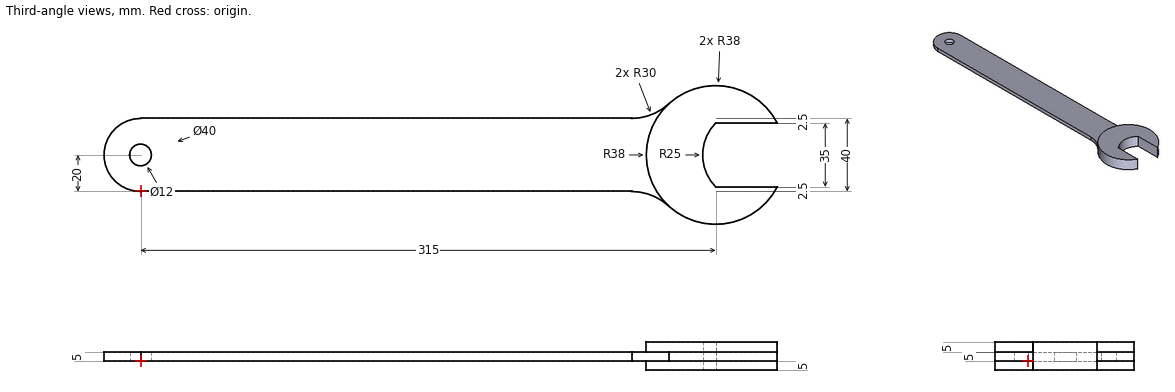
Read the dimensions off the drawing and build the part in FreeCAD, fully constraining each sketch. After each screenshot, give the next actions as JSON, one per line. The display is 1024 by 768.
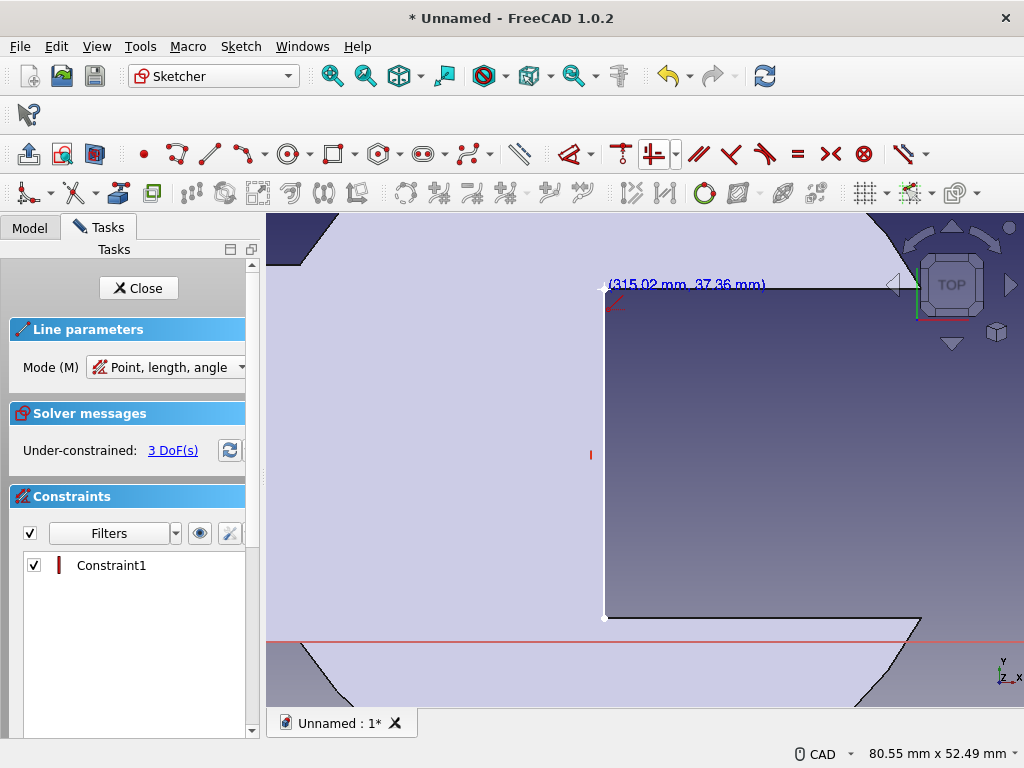
{"action": "left_click", "coordinate": [242, 154]}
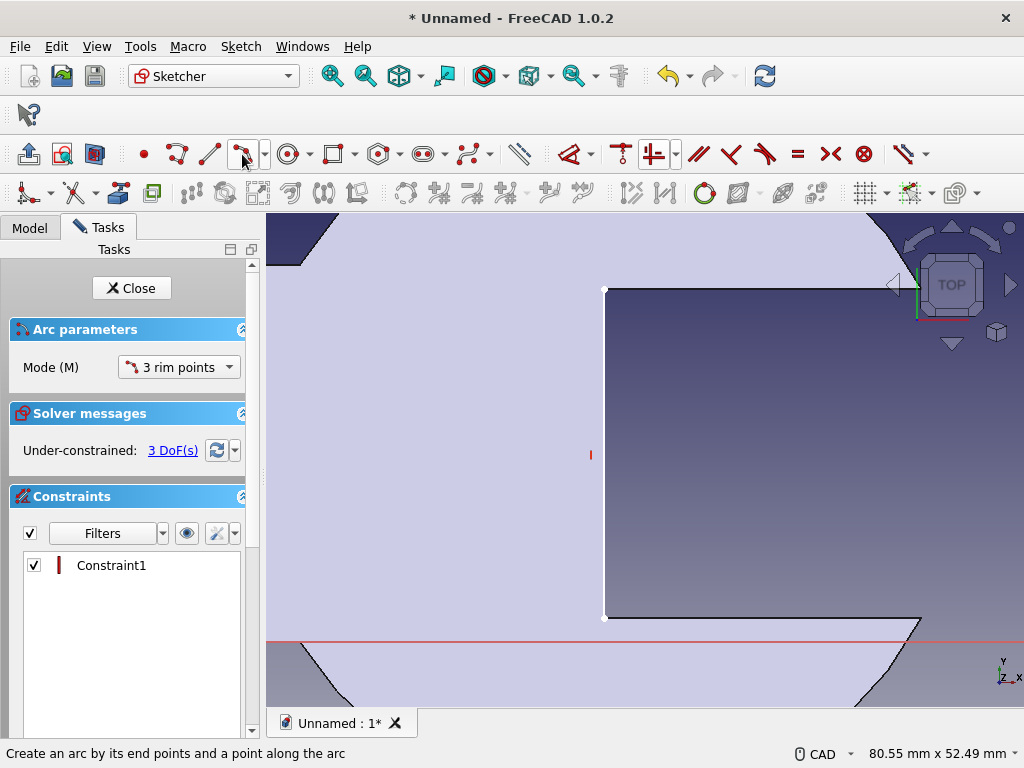
{"action": "left_click", "coordinate": [604, 290]}
{"action": "left_click", "coordinate": [604, 619]}
{"action": "left_click", "coordinate": [537, 453]}
{"action": "key", "text": "Escape"}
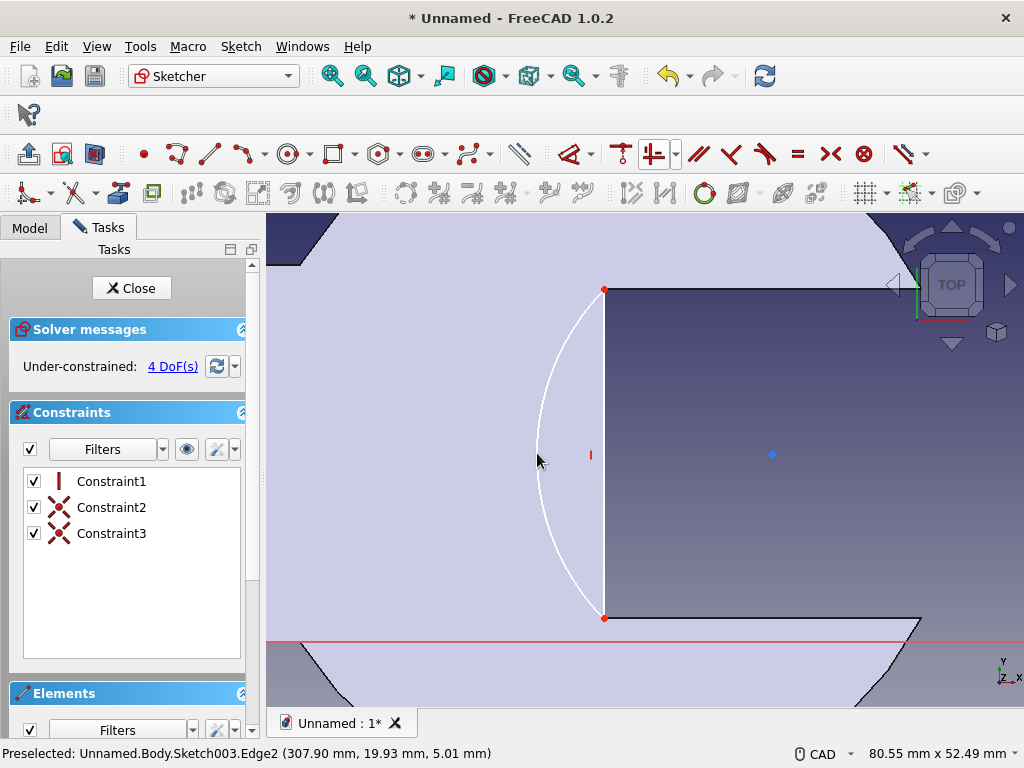
{"action": "left_click", "coordinate": [568, 154]}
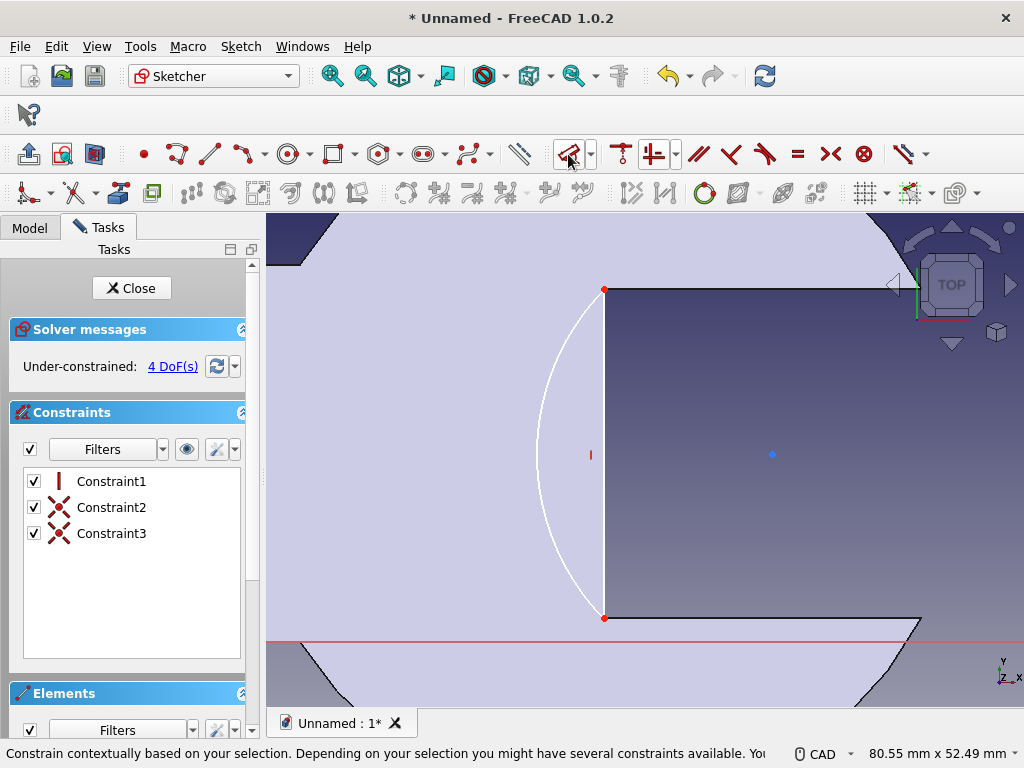
{"action": "left_click", "coordinate": [548, 383]}
{"action": "left_click", "coordinate": [518, 373]}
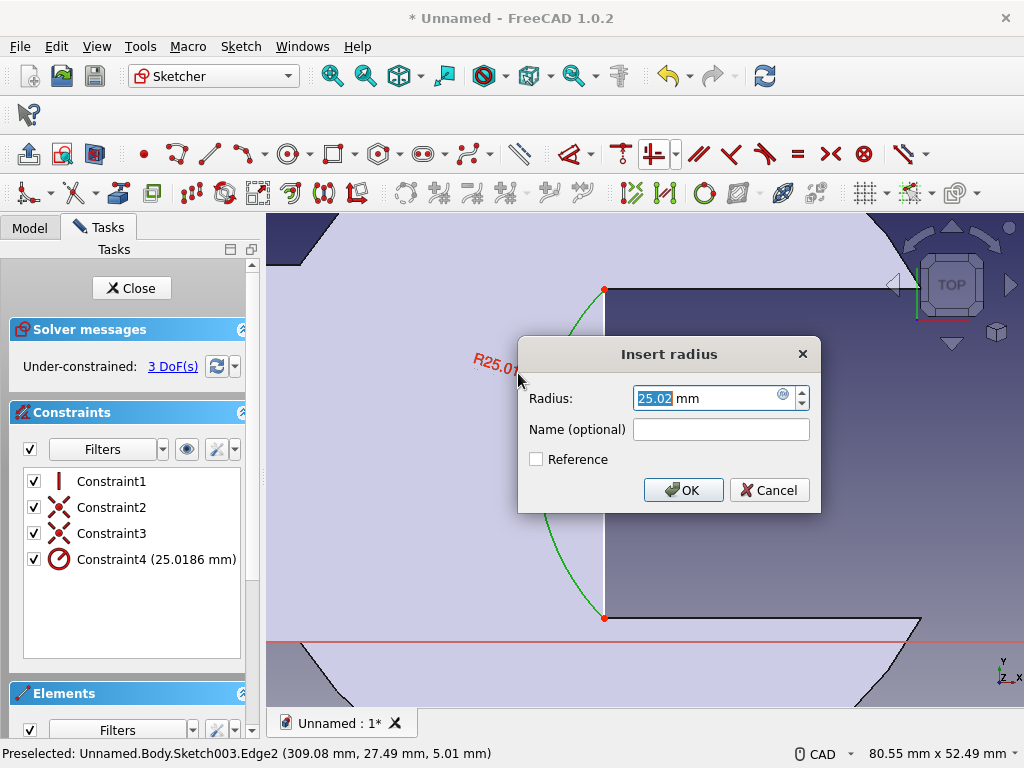
{"action": "type", "text": "25"}
{"action": "key", "text": "Return"}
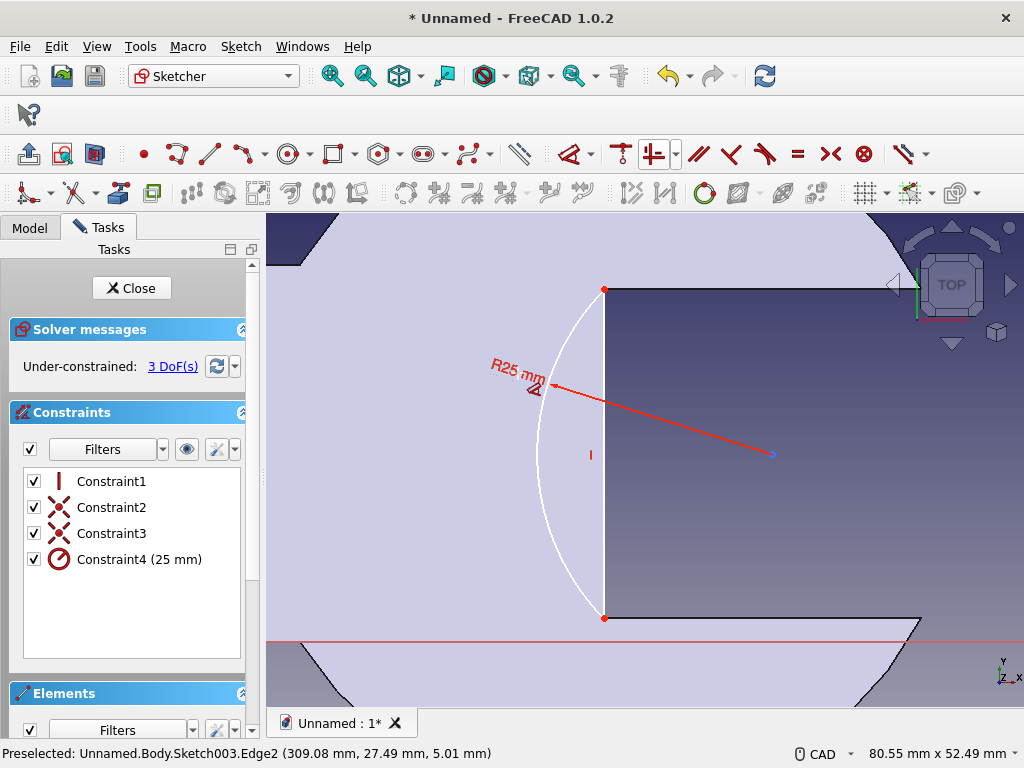
{"action": "left_click", "coordinate": [604, 520]}
{"action": "left_click", "coordinate": [638, 454]}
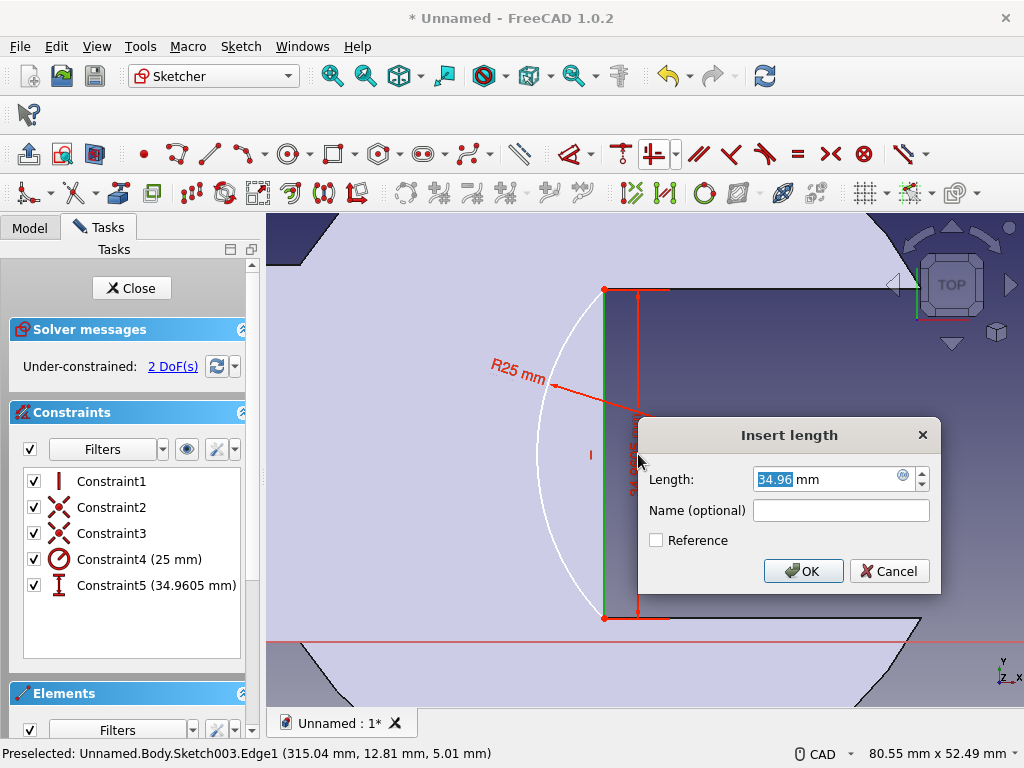
{"action": "type", "text": "35"}
{"action": "key", "text": "Return"}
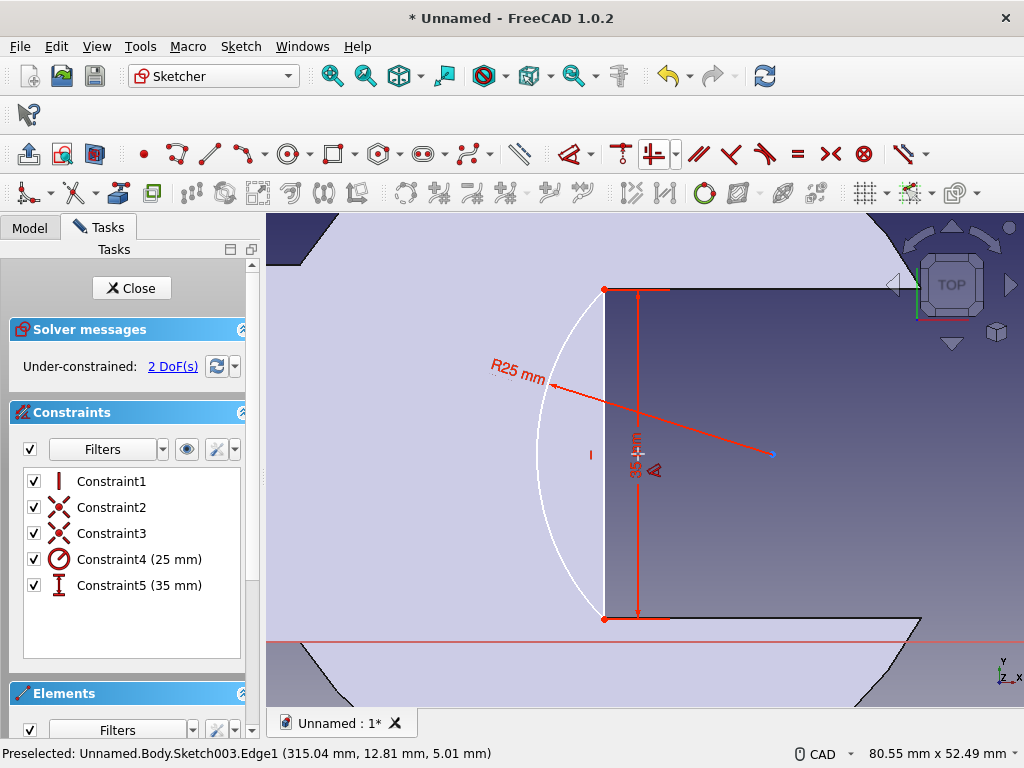
{"action": "left_click", "coordinate": [772, 455]}
{"action": "left_click", "coordinate": [806, 548]}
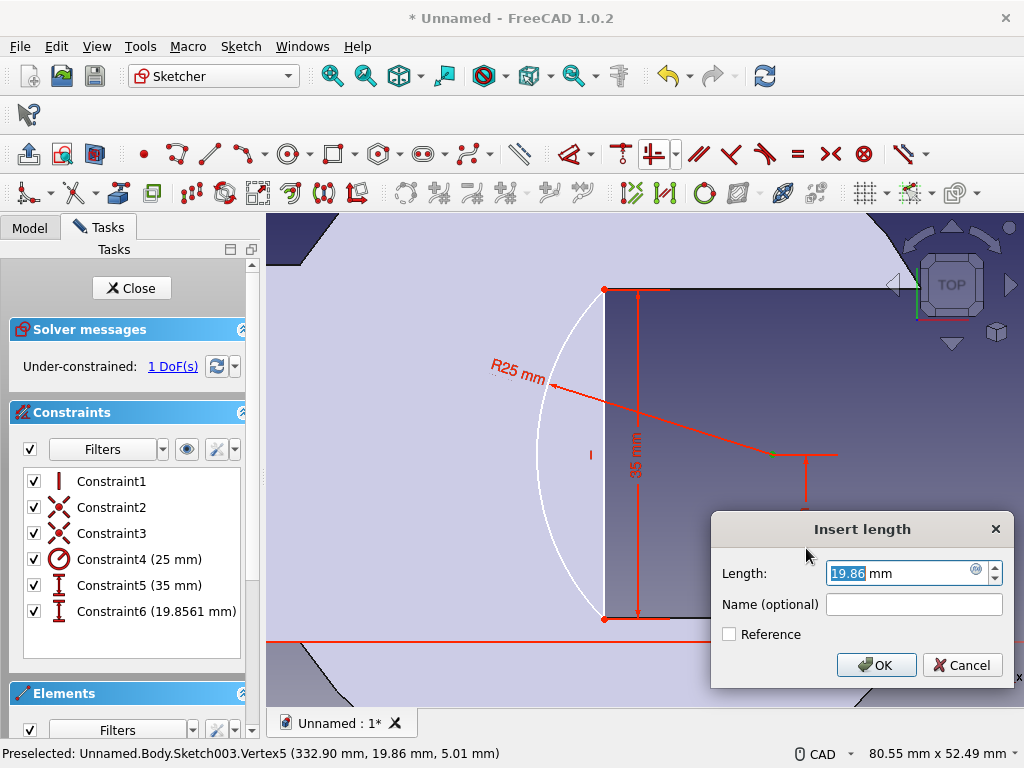
{"action": "type", "text": "20"}
{"action": "key", "text": "Return"}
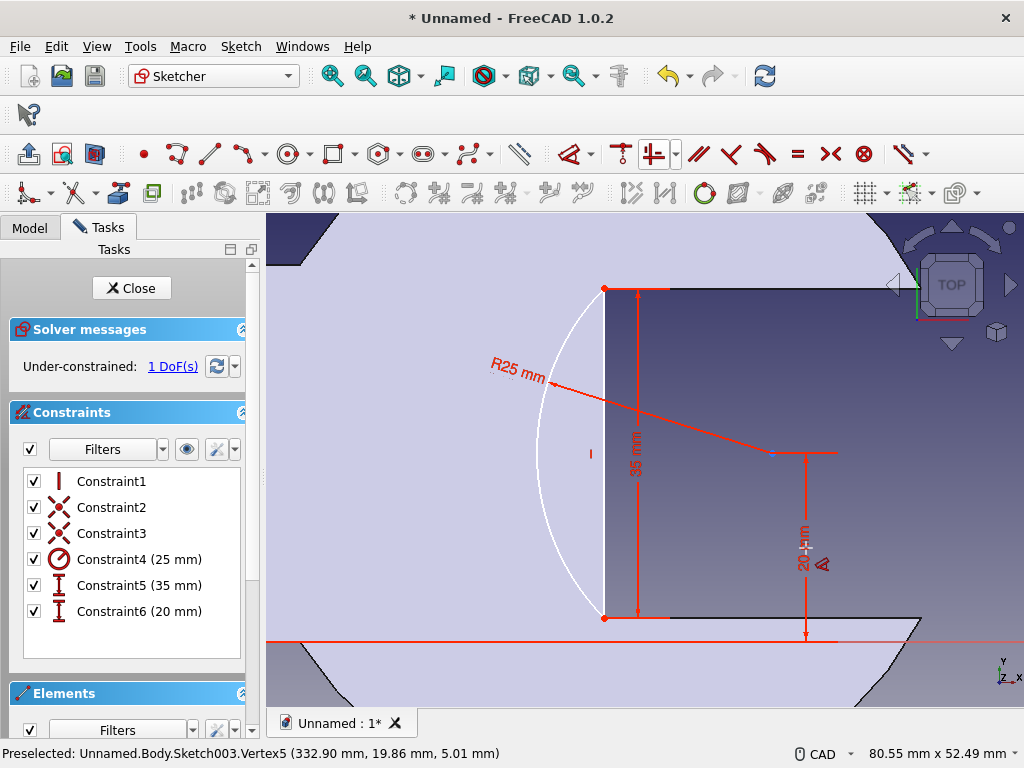
{"action": "left_click", "coordinate": [604, 618]}
{"action": "left_click", "coordinate": [449, 676]}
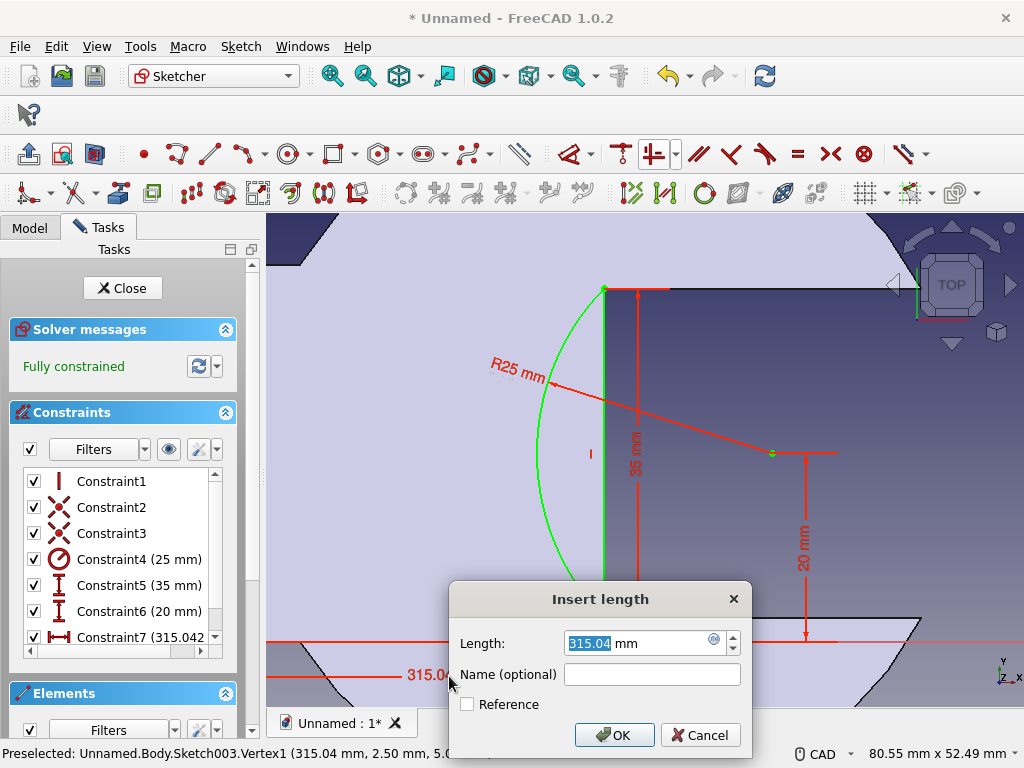
{"action": "type", "text": "315"}
{"action": "key", "text": "Return"}
{"action": "key", "text": "Escape"}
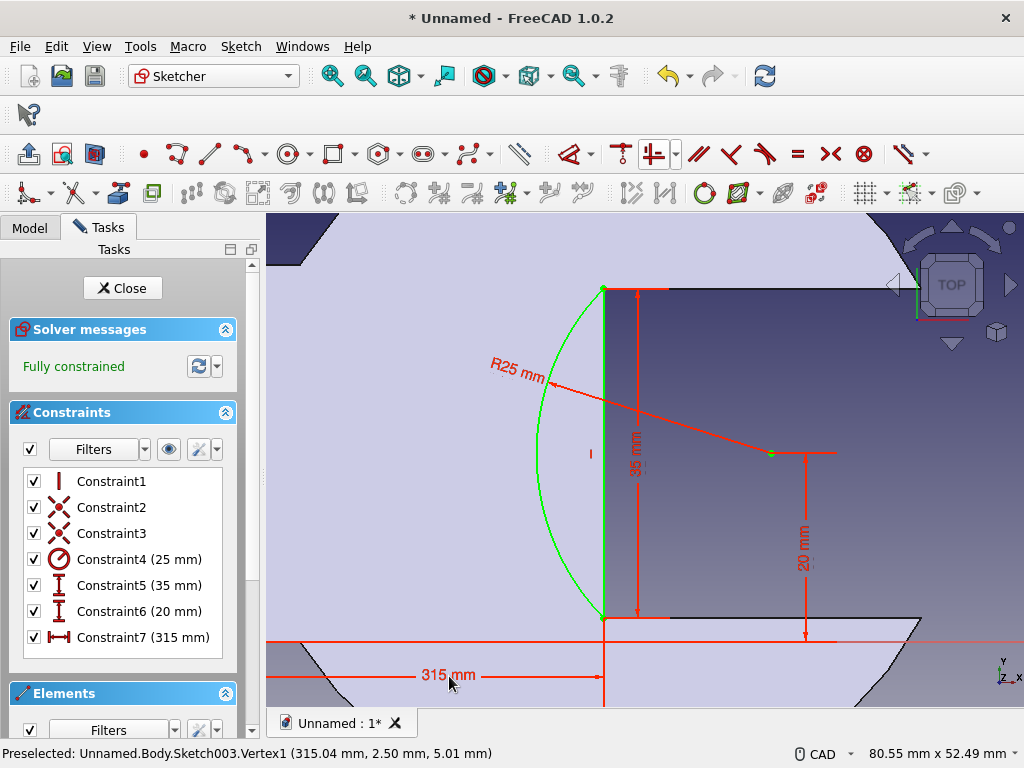
{"action": "left_click", "coordinate": [123, 288]}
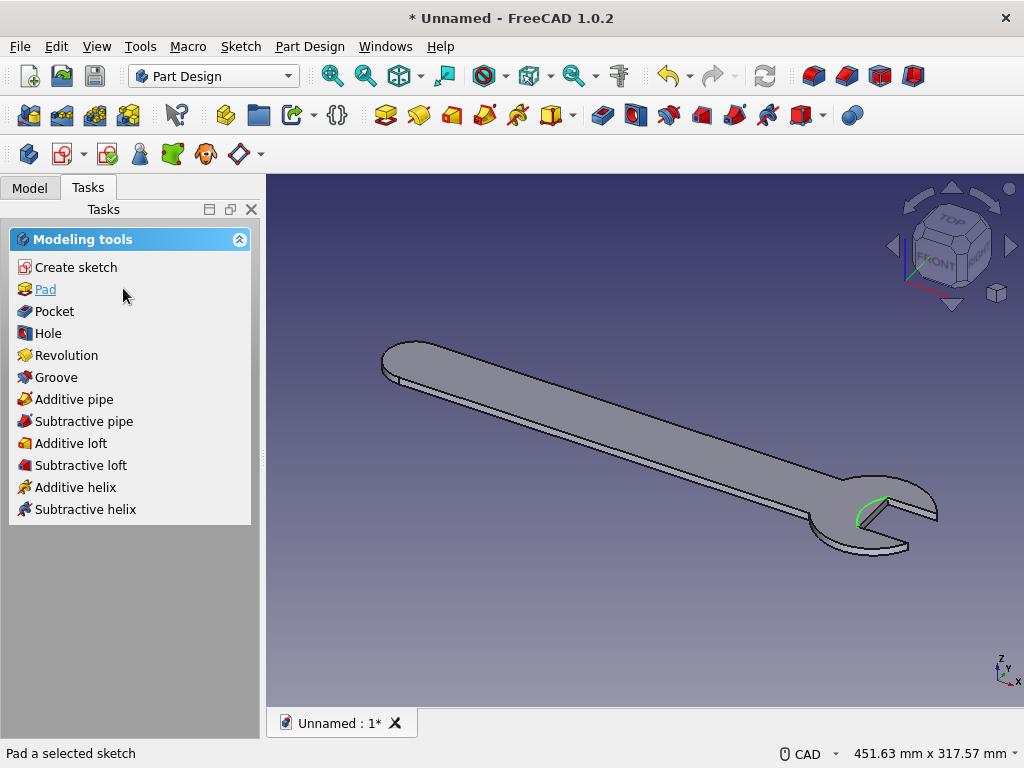
{"action": "left_click", "coordinate": [603, 116]}